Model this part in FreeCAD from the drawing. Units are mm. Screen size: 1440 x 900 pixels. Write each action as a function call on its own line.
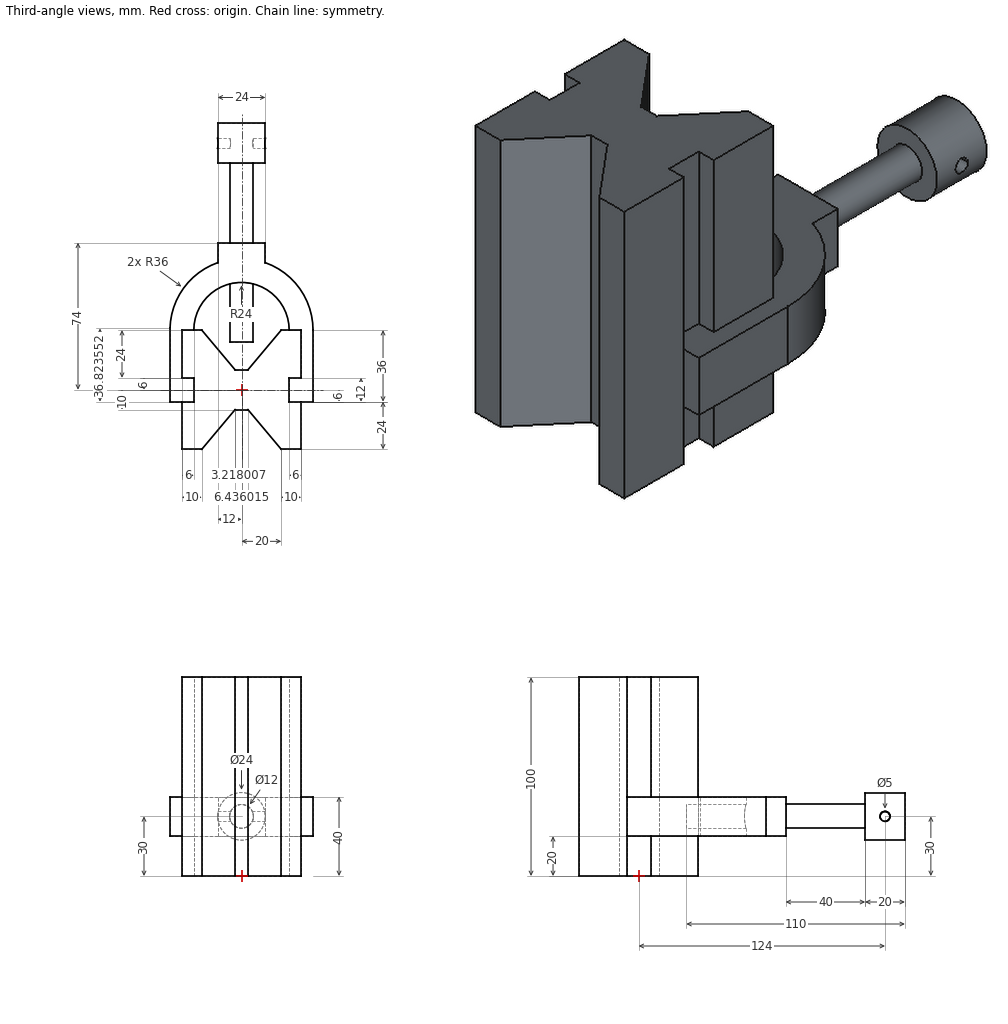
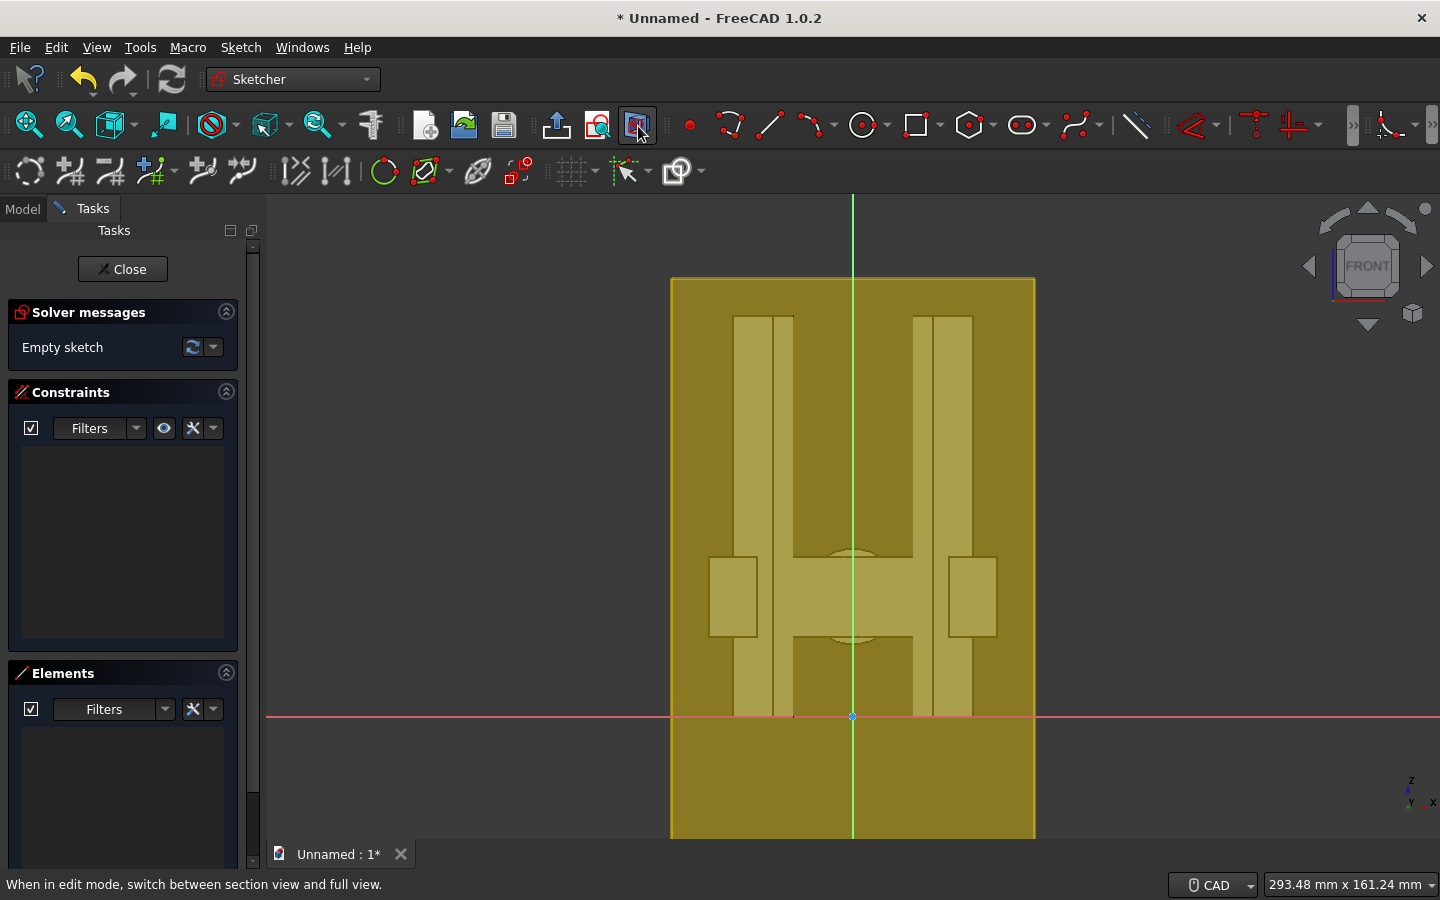
scroll(862, 606, up, 11)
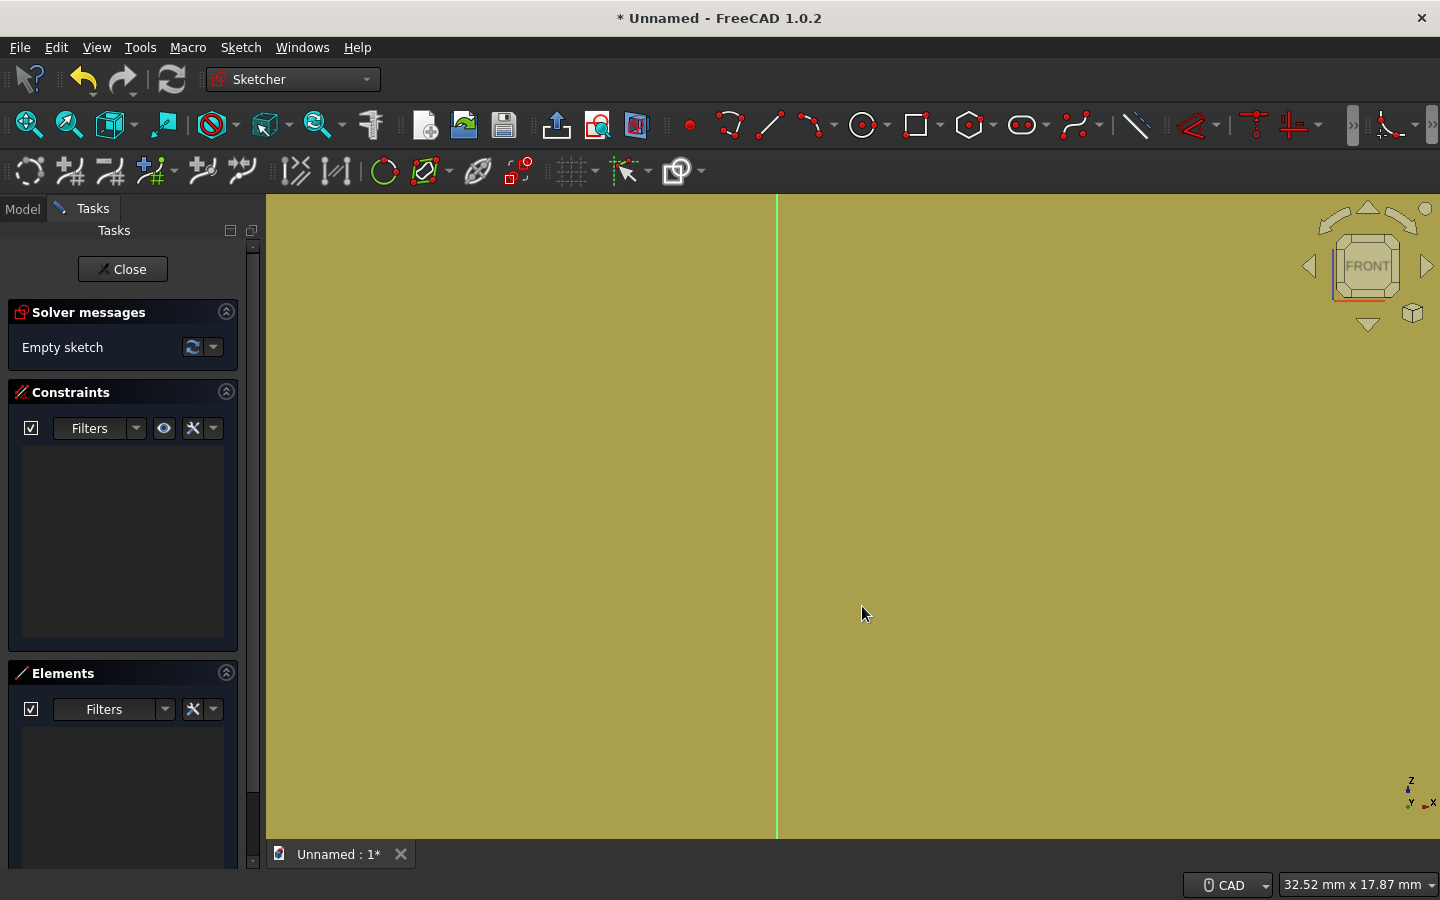
click(864, 126)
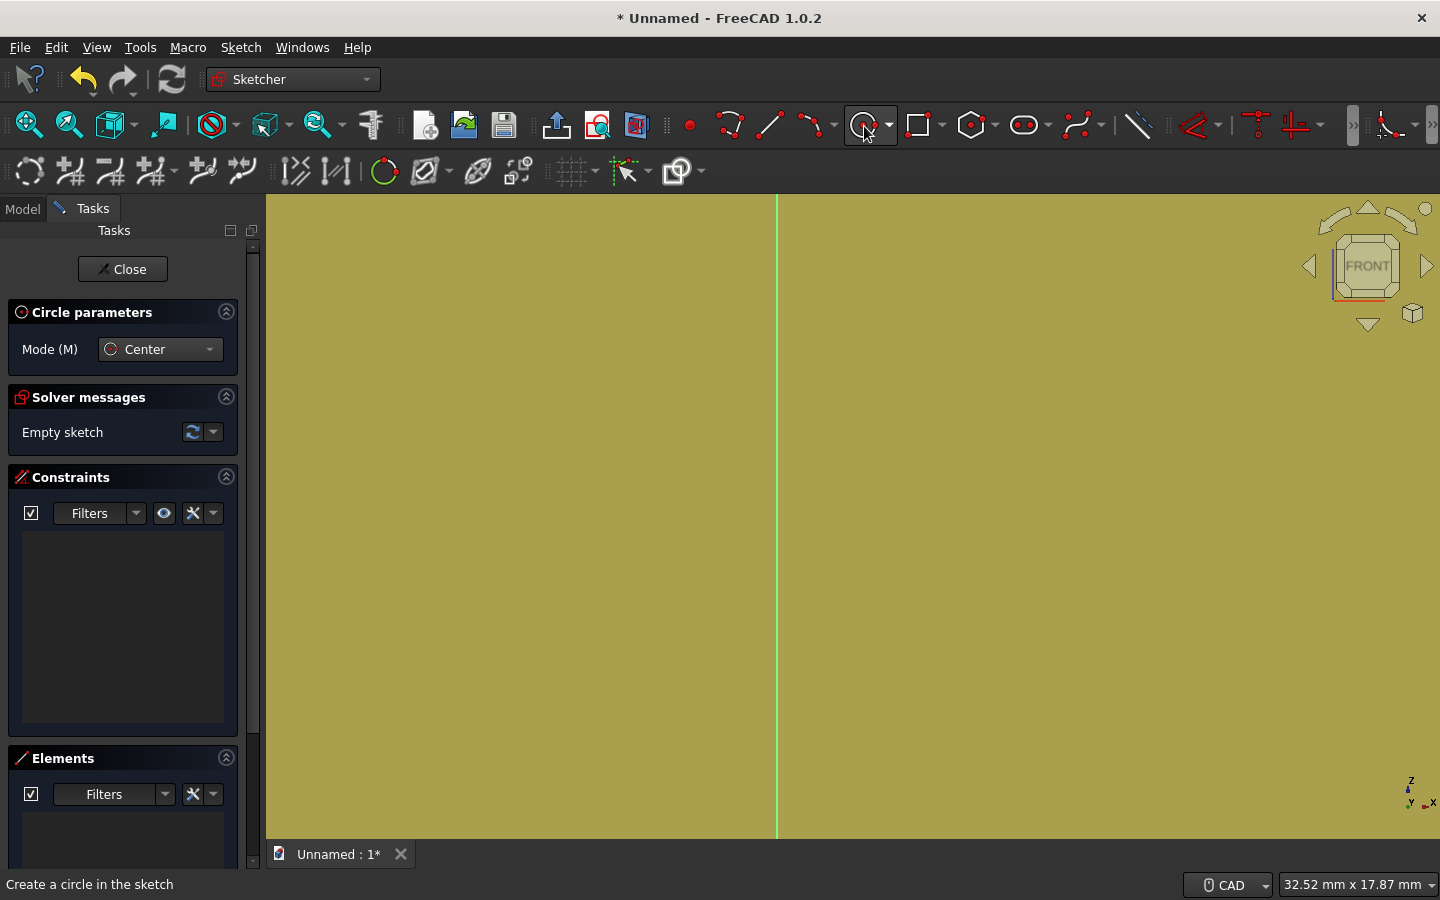
click(777, 515)
move(930, 362)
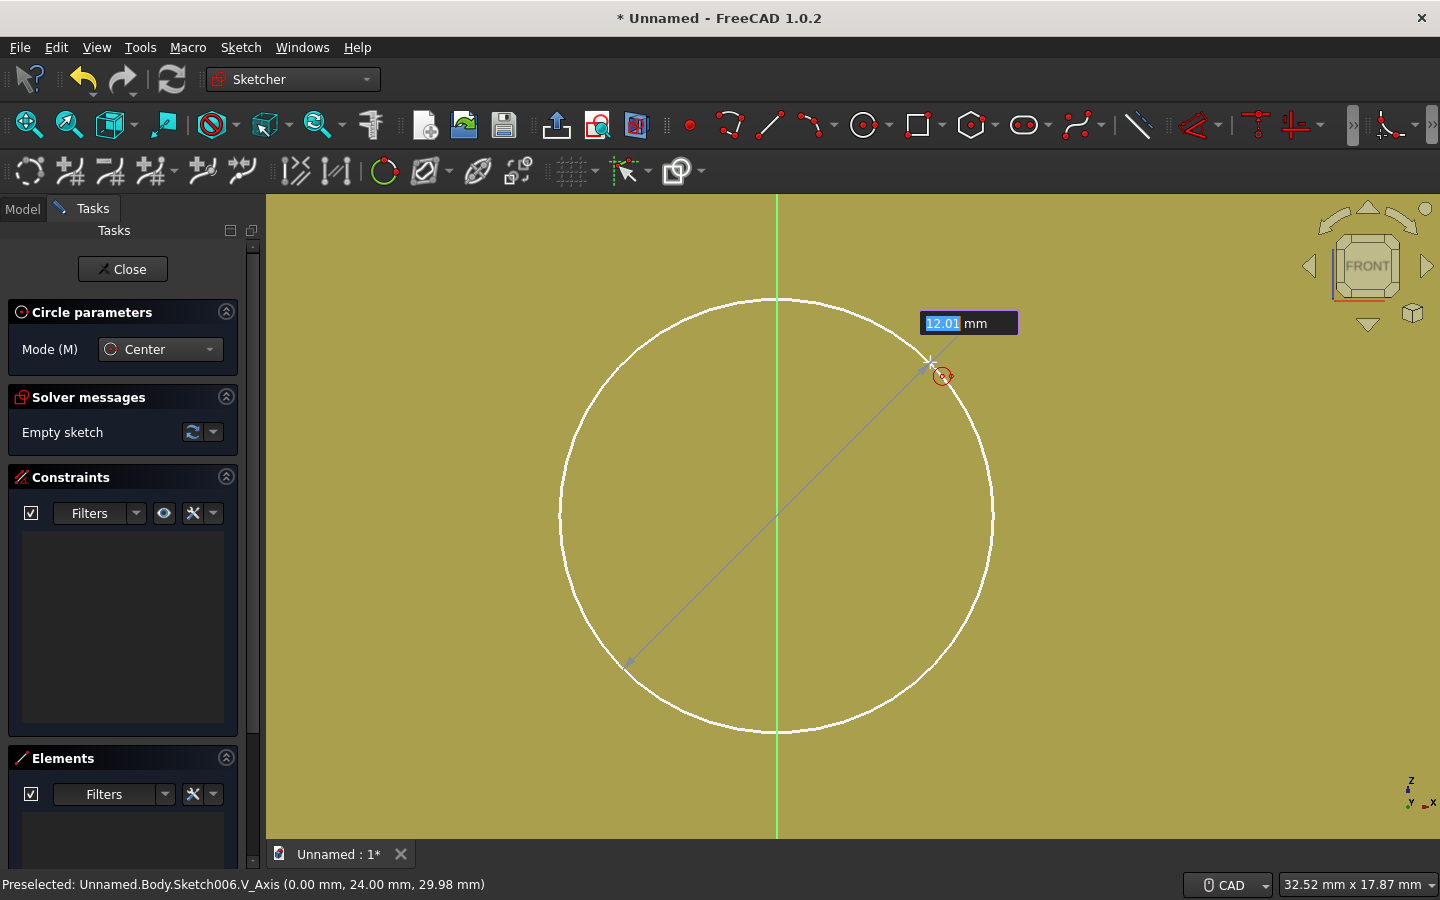
text(12)
key(Return)
key(Escape)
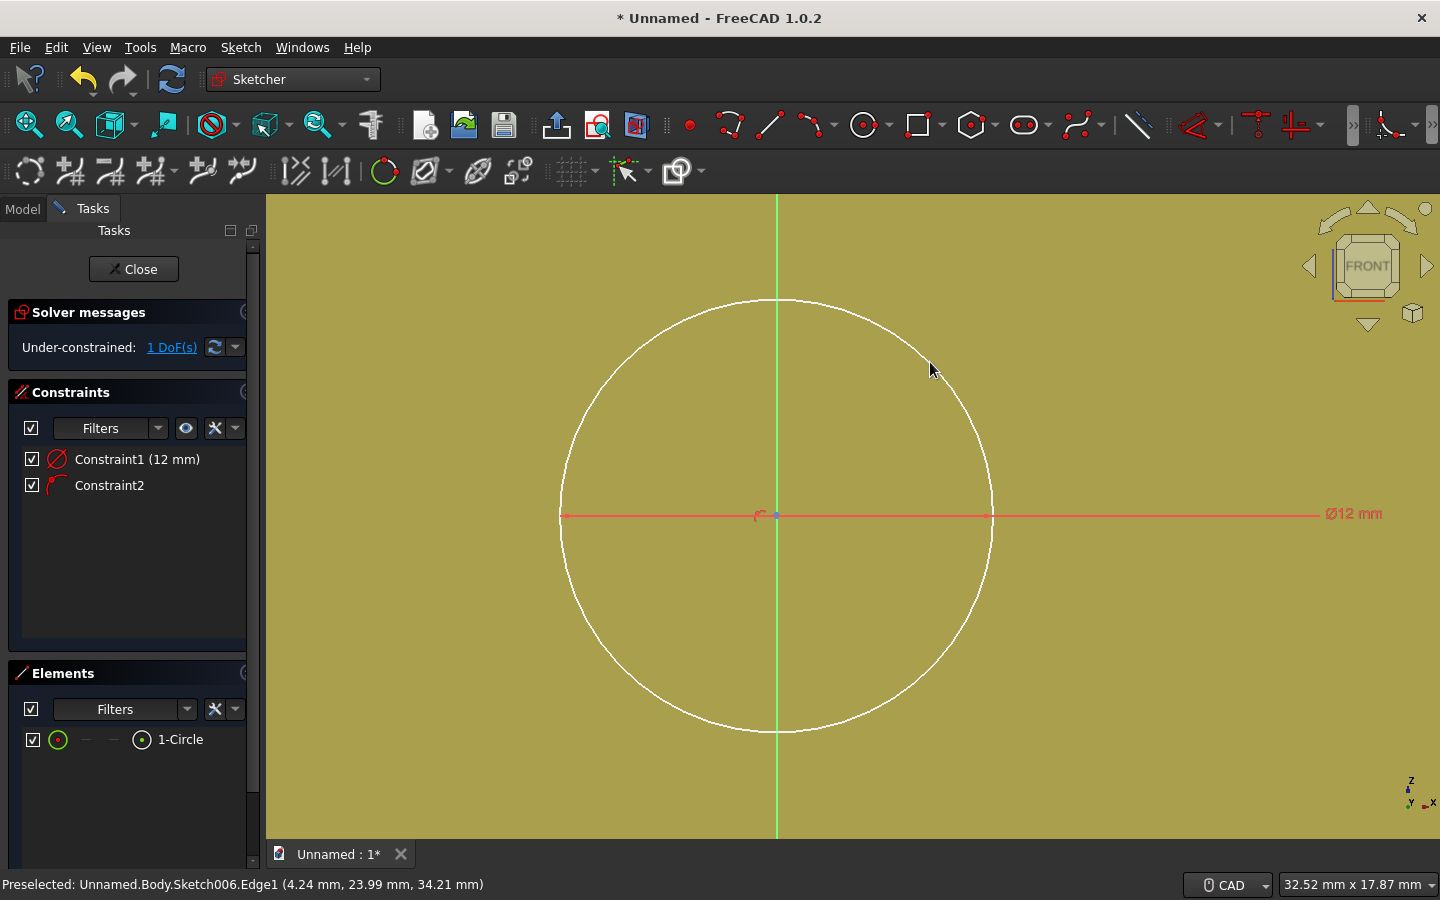
key(d)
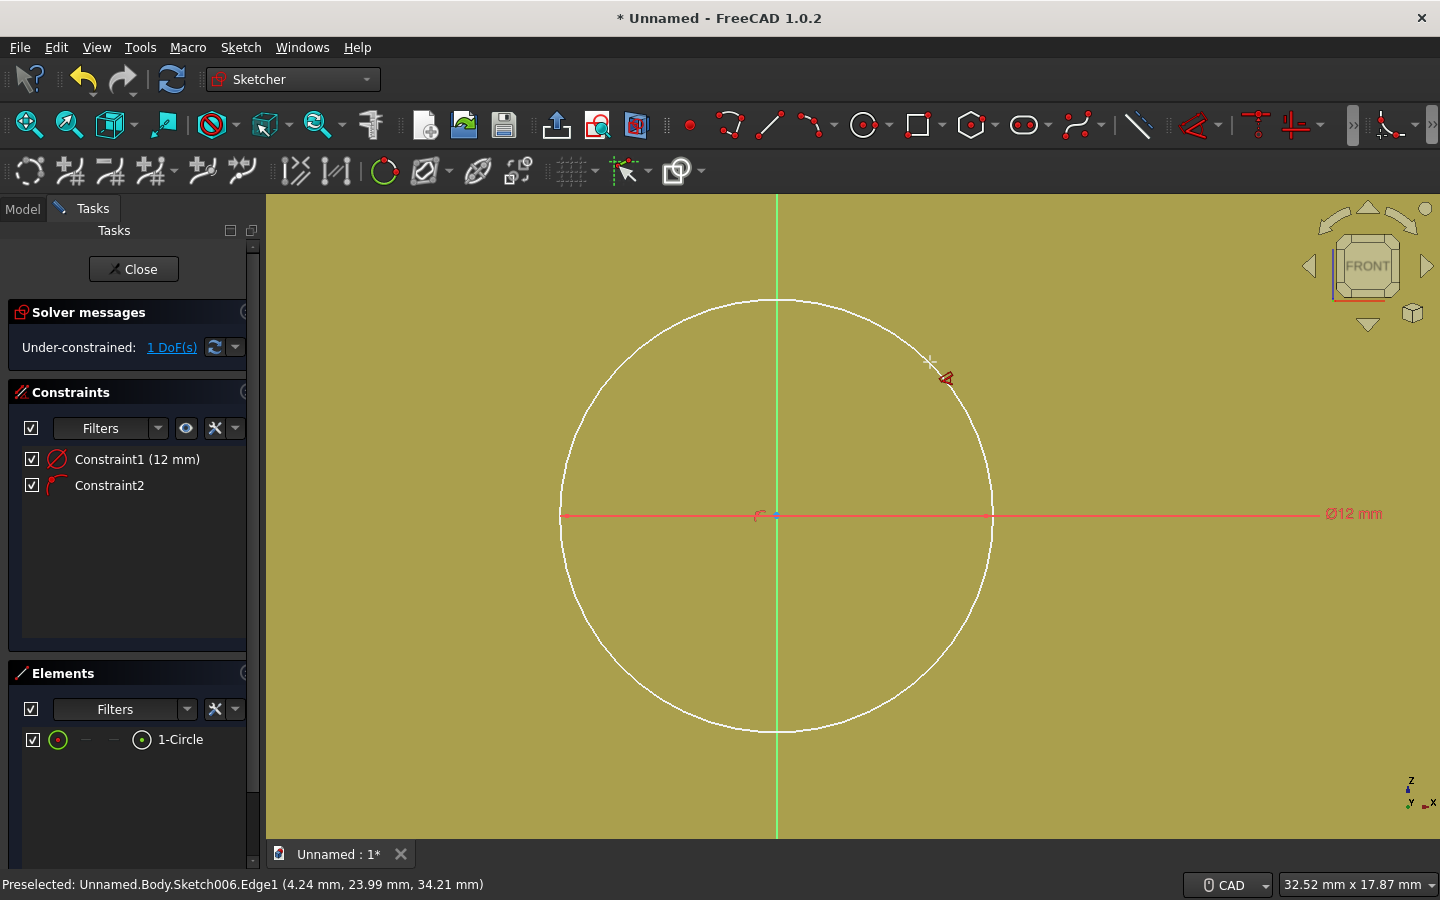
click(777, 516)
click(811, 664)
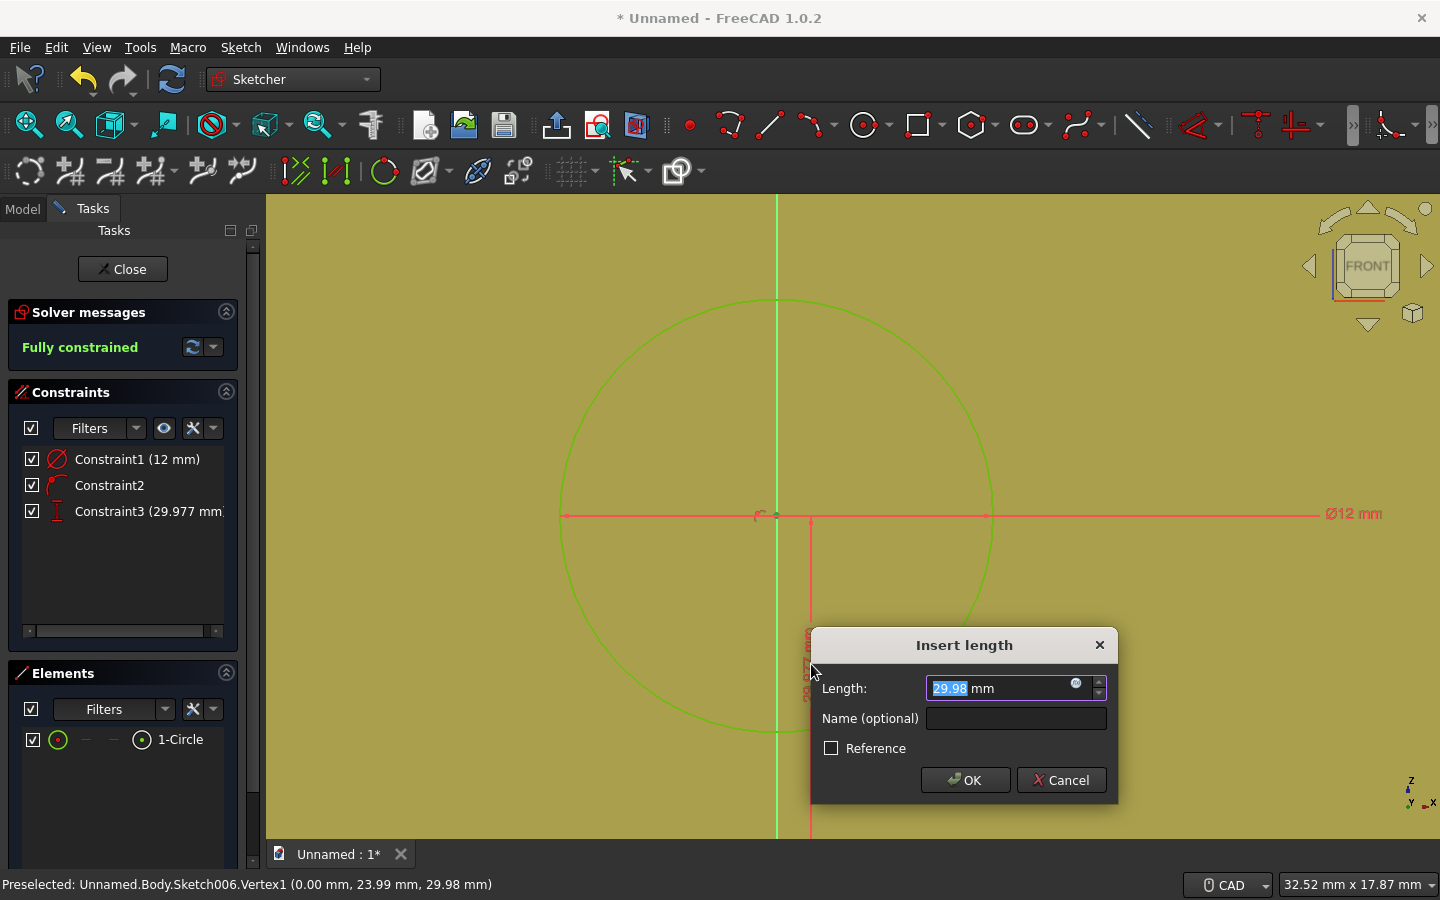
text(30)
key(Return)
key(Escape)